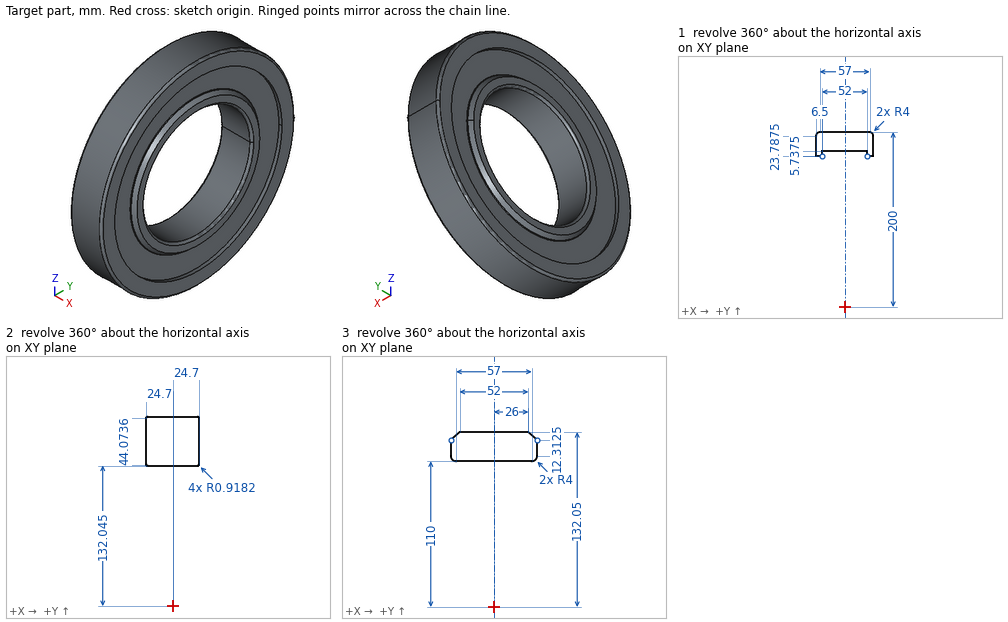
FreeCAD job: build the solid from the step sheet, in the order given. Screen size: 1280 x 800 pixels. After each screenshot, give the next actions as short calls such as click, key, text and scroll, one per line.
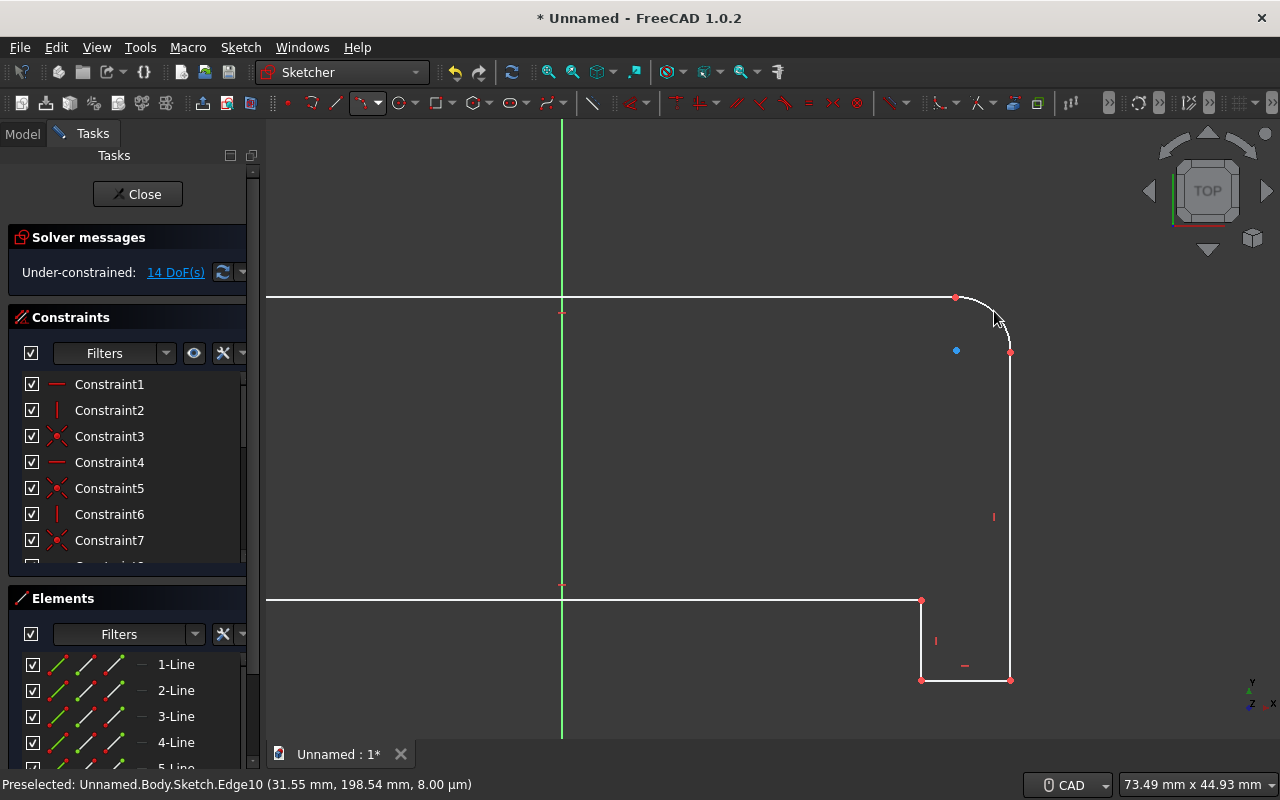
click(719, 297)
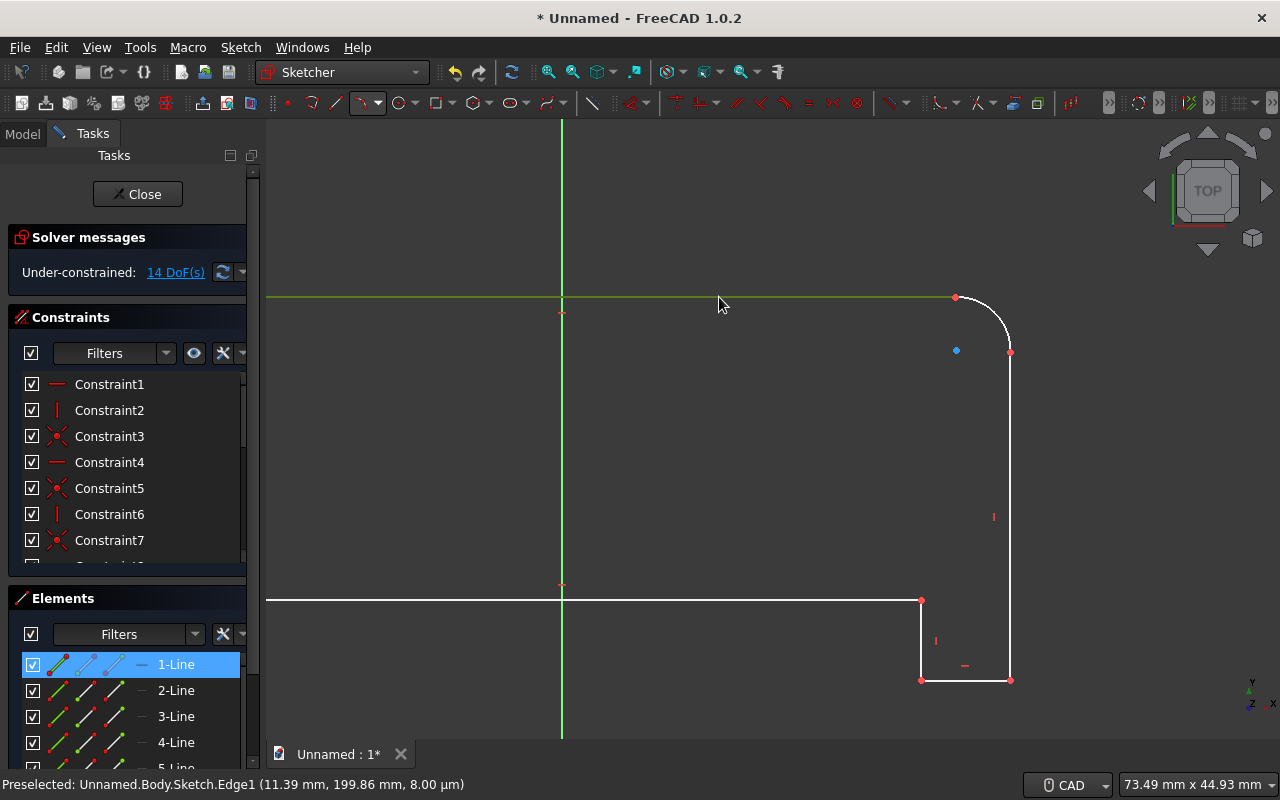
scroll(995, 311, down, 2)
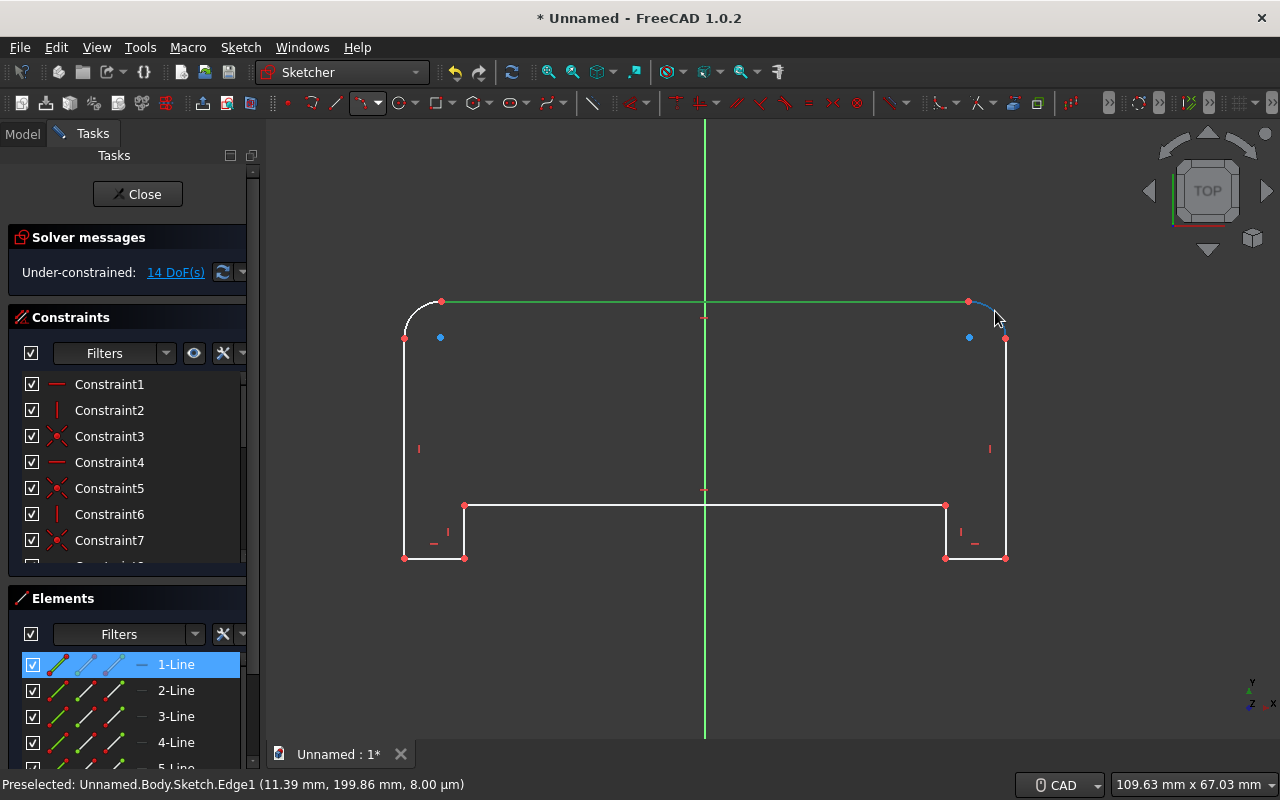
click(424, 306)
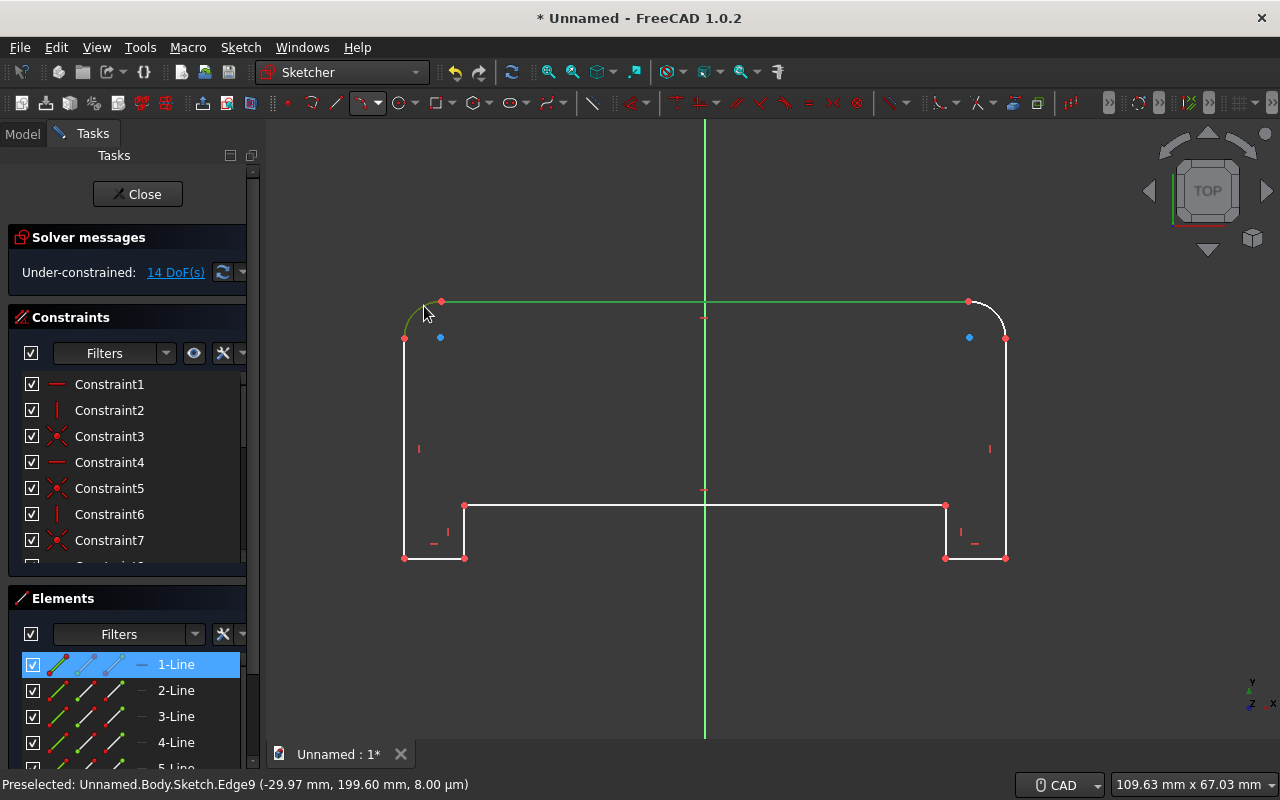
click(786, 104)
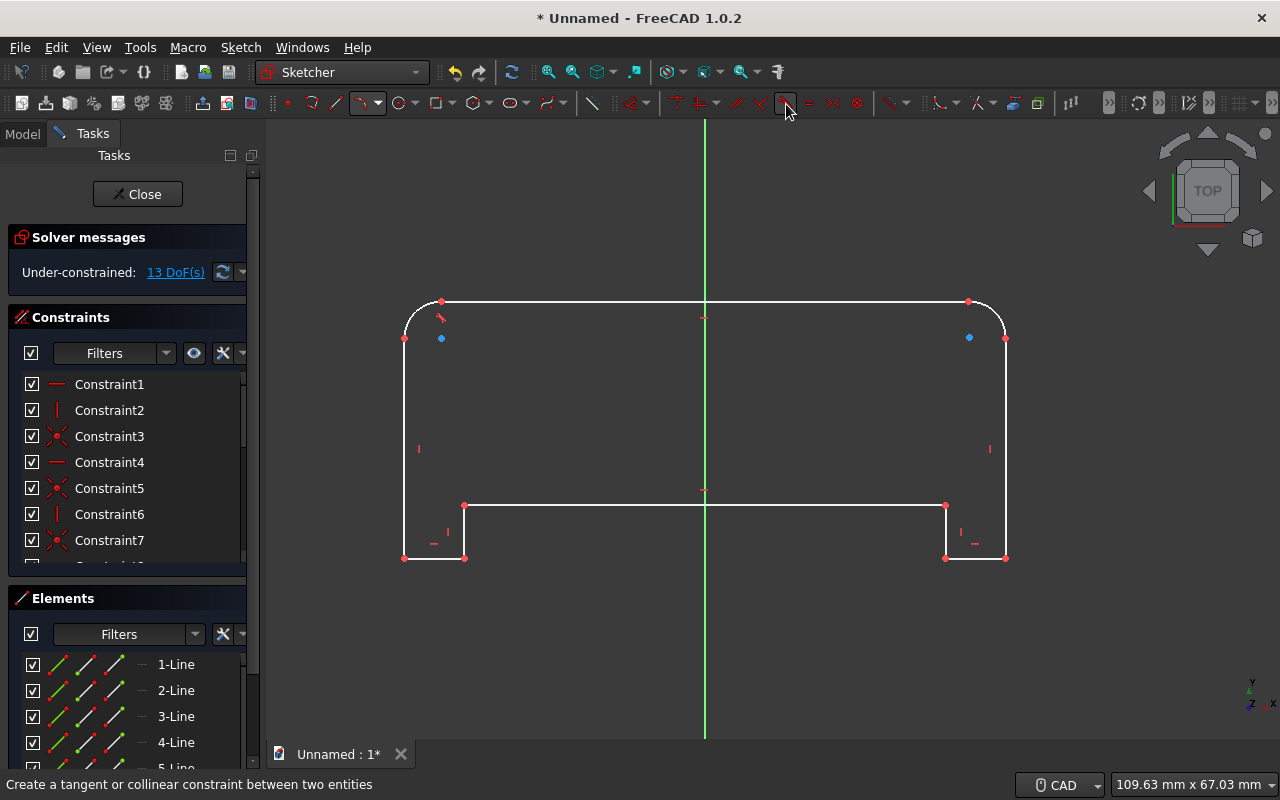
click(810, 302)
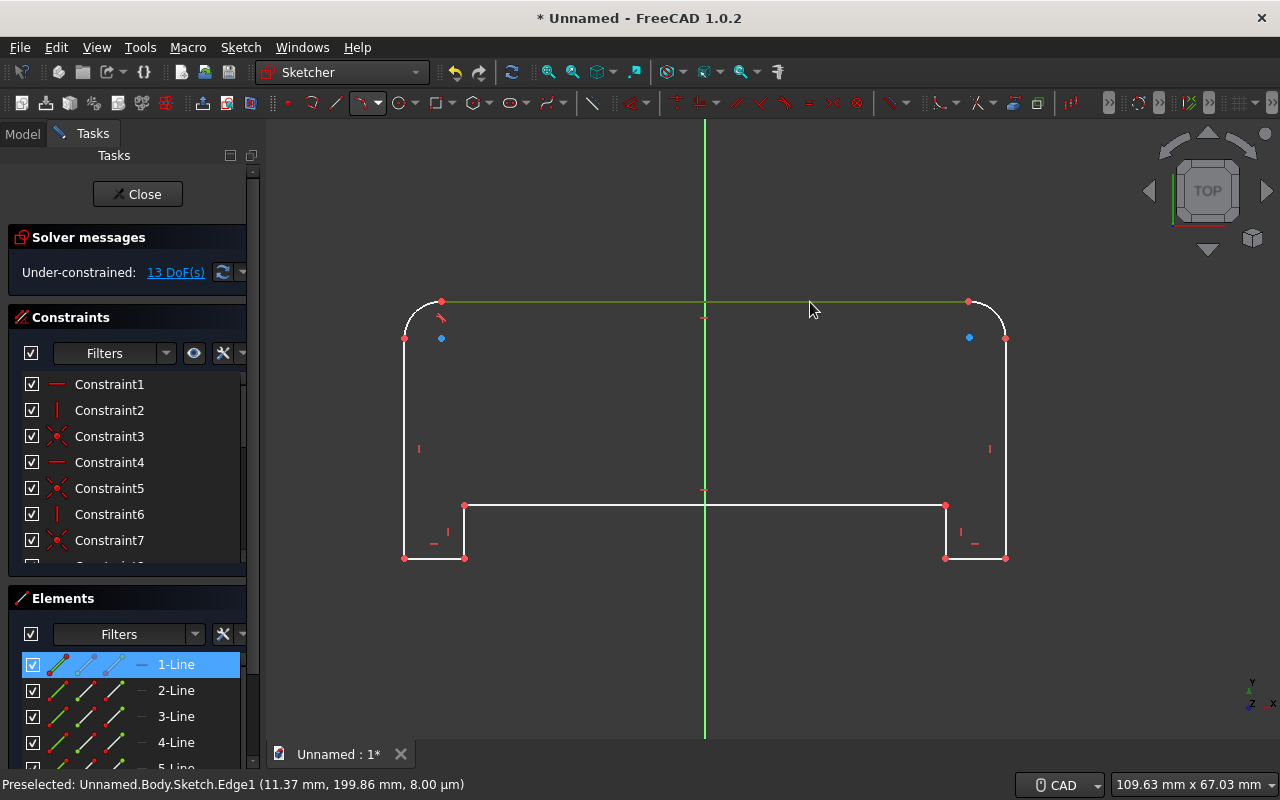
click(1002, 322)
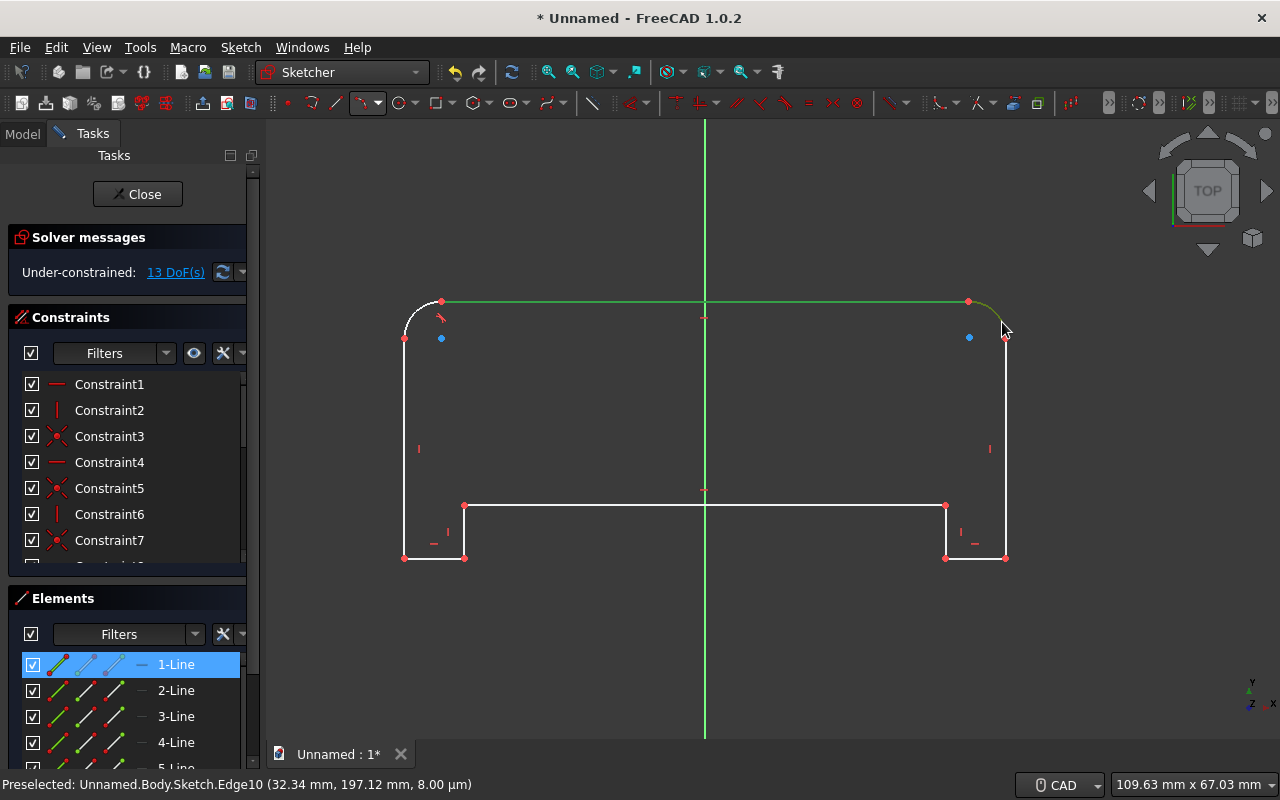
click(786, 104)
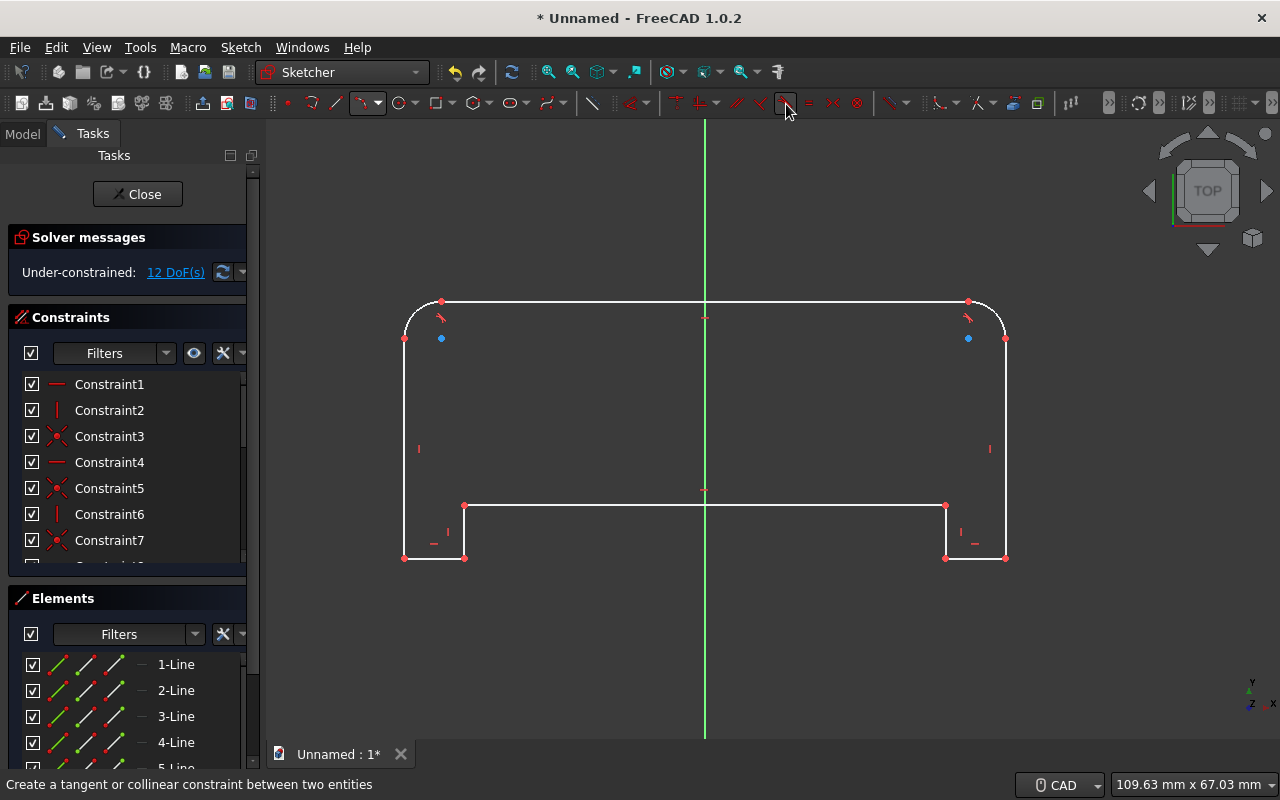
click(404, 405)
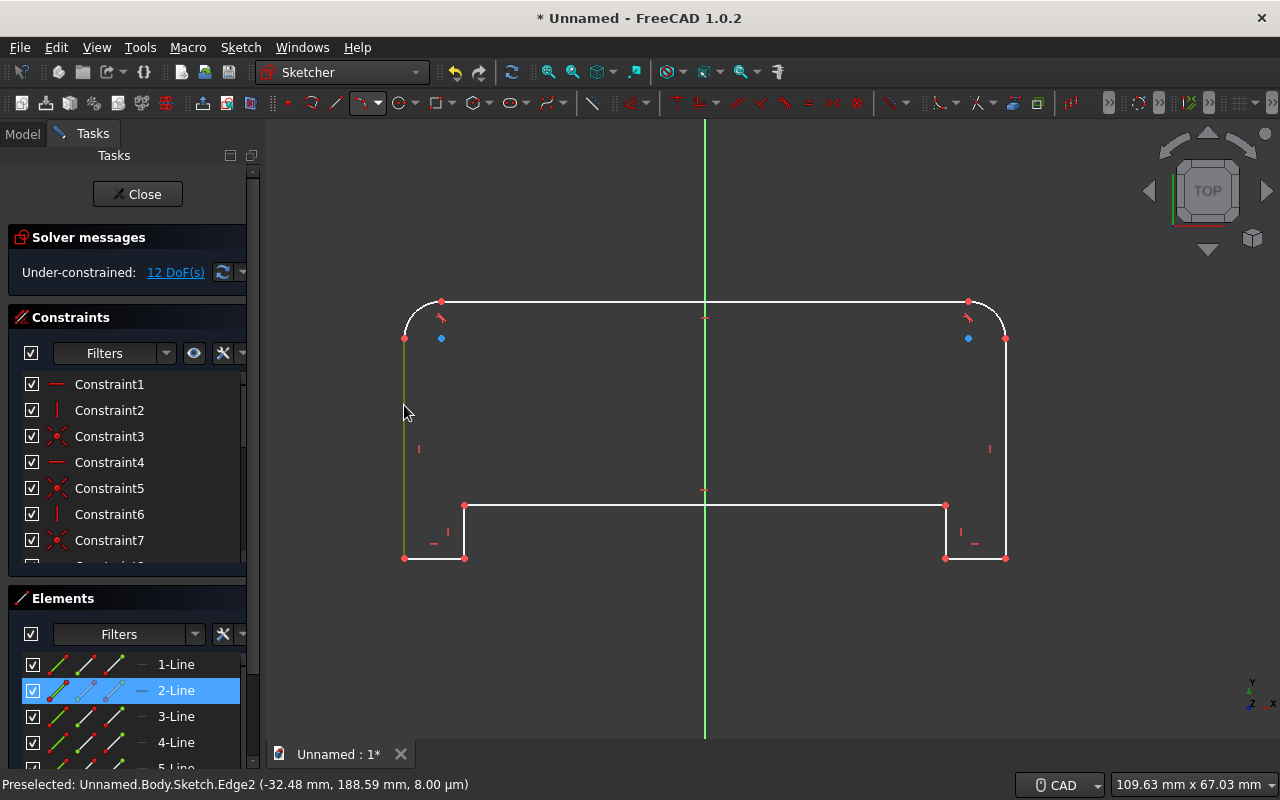
click(425, 306)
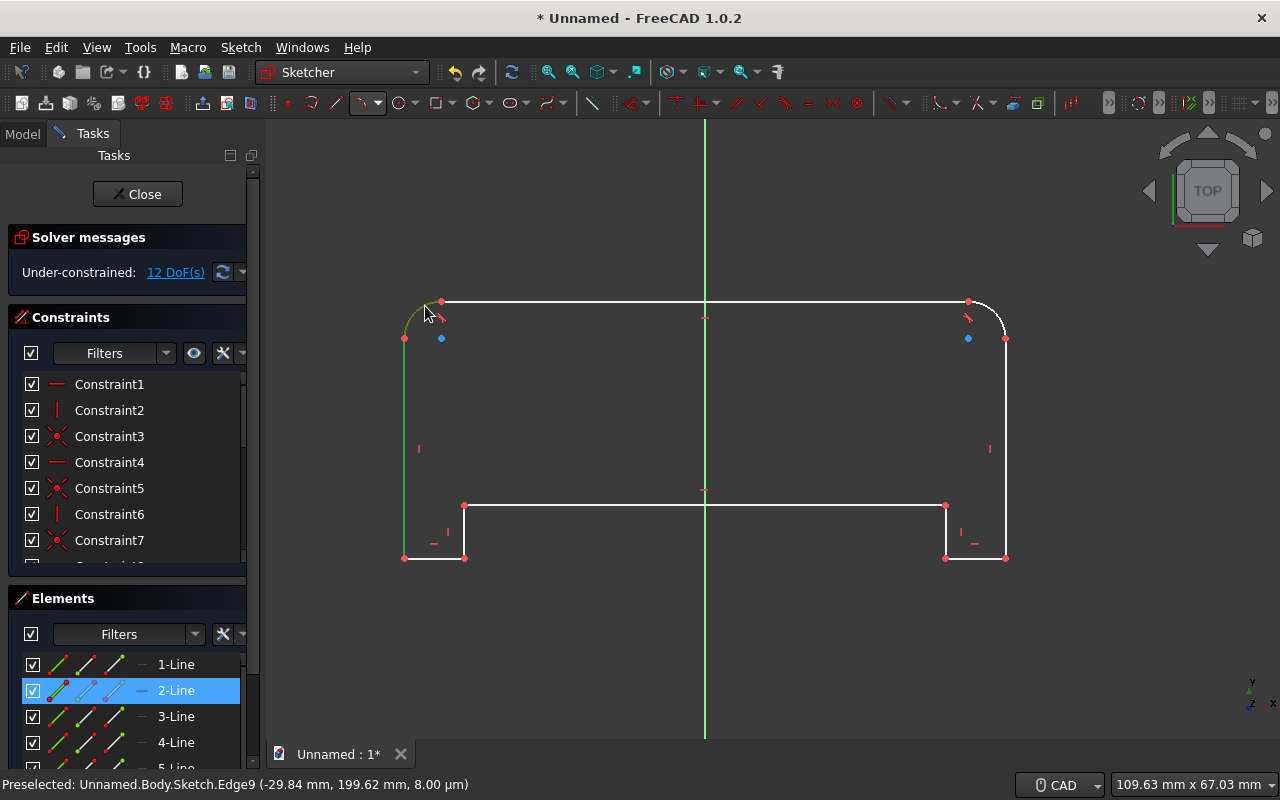
click(786, 104)